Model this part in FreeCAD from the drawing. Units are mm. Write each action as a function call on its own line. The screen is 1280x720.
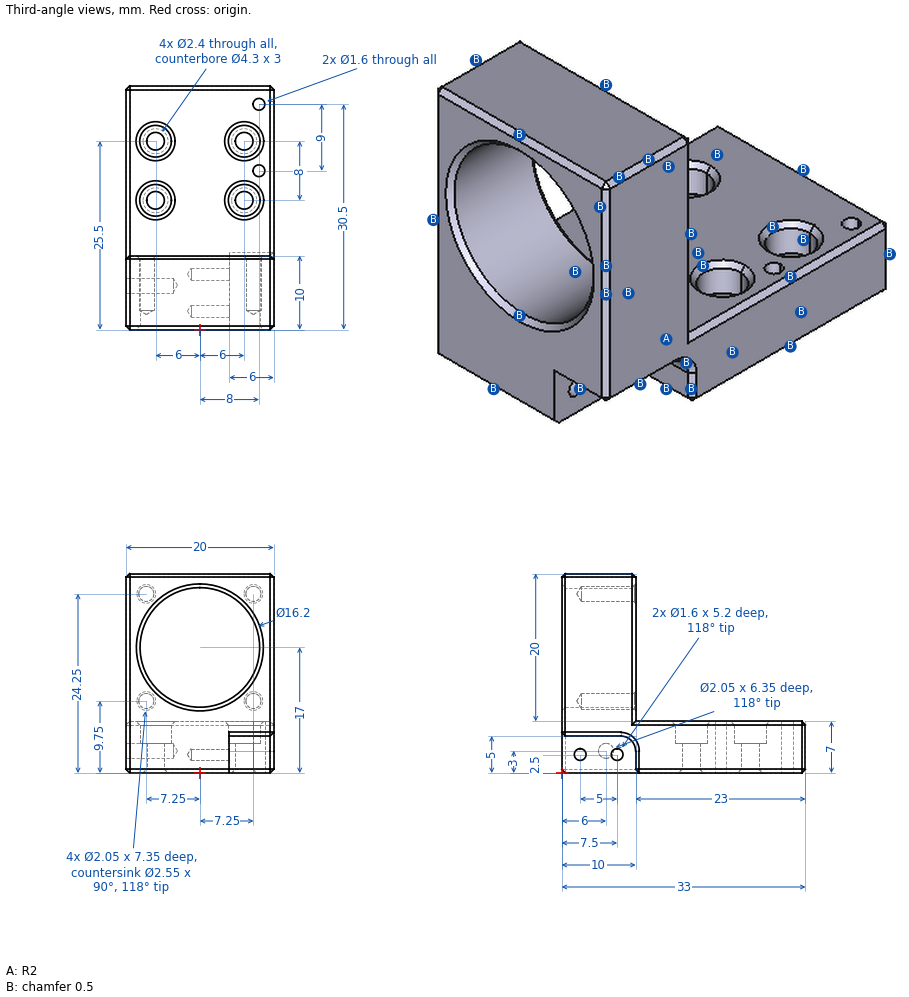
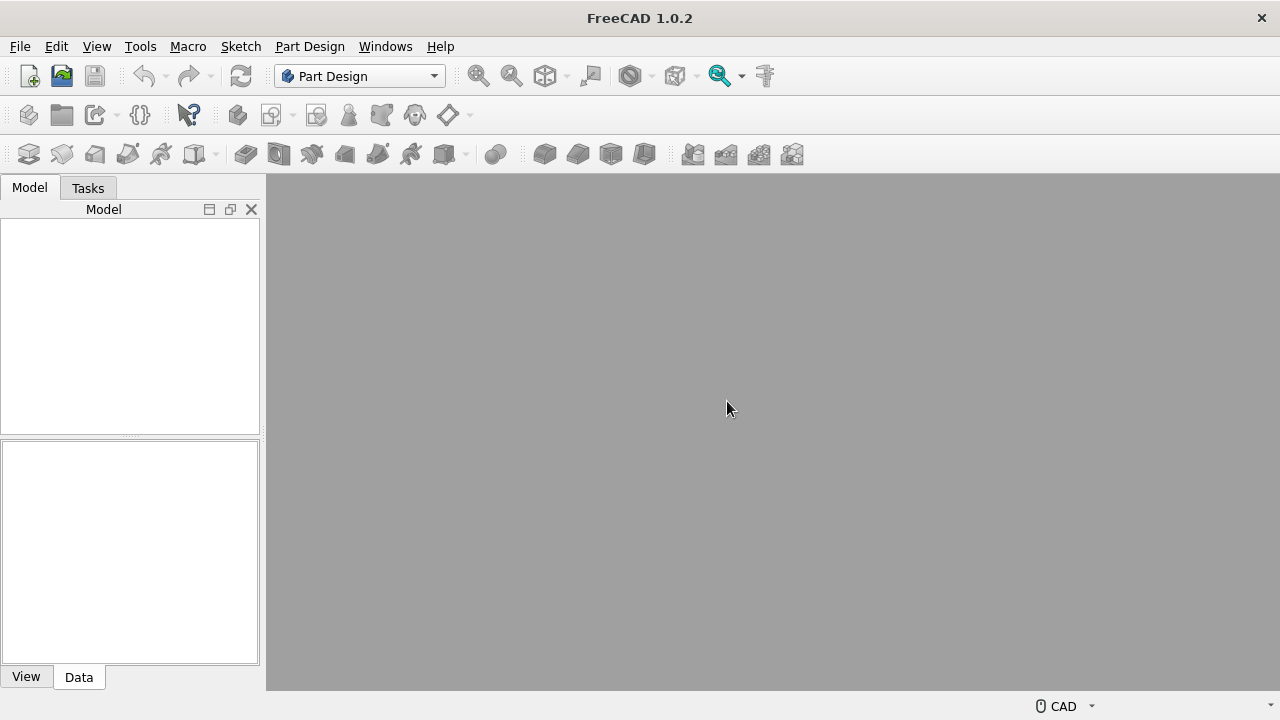
click(29, 76)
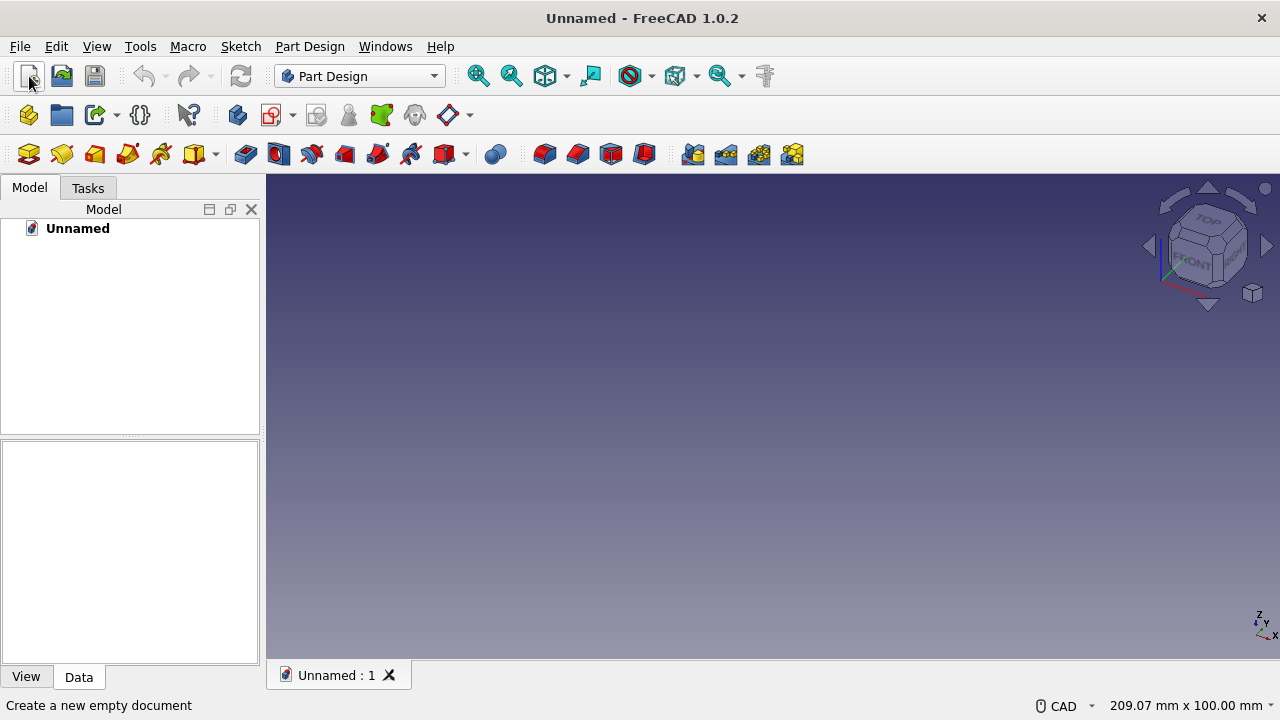
click(270, 116)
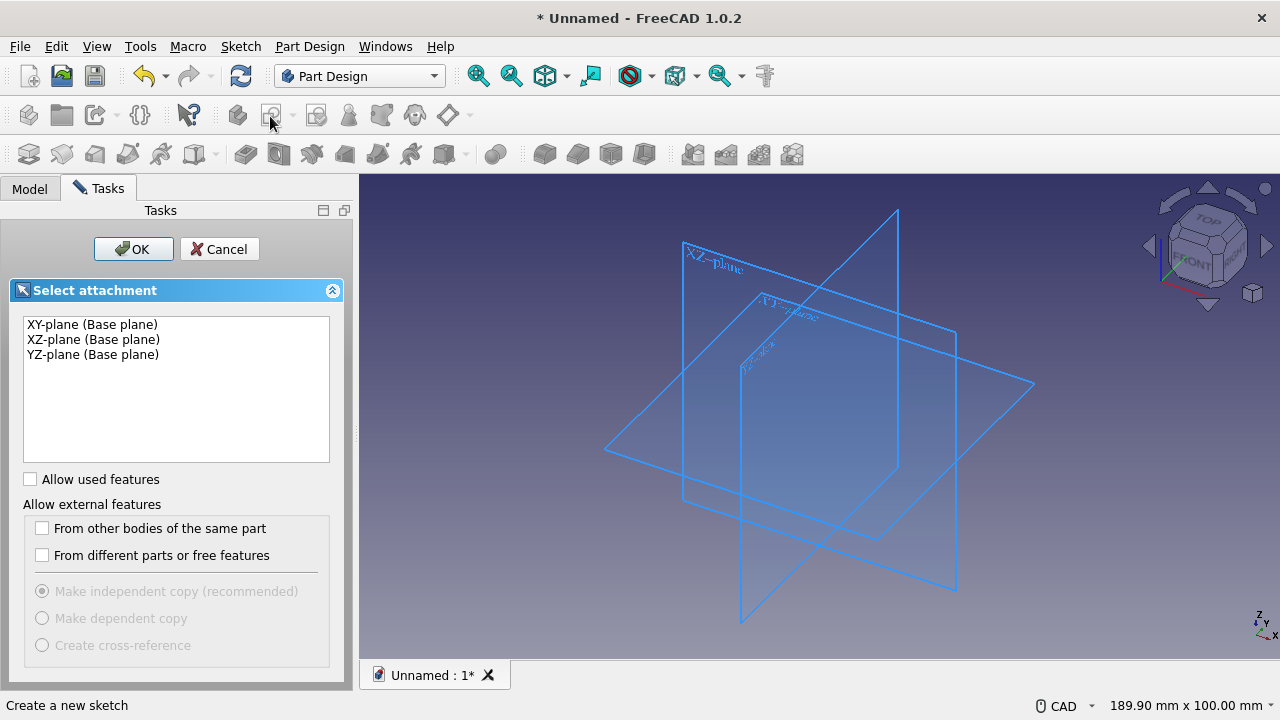
click(84, 354)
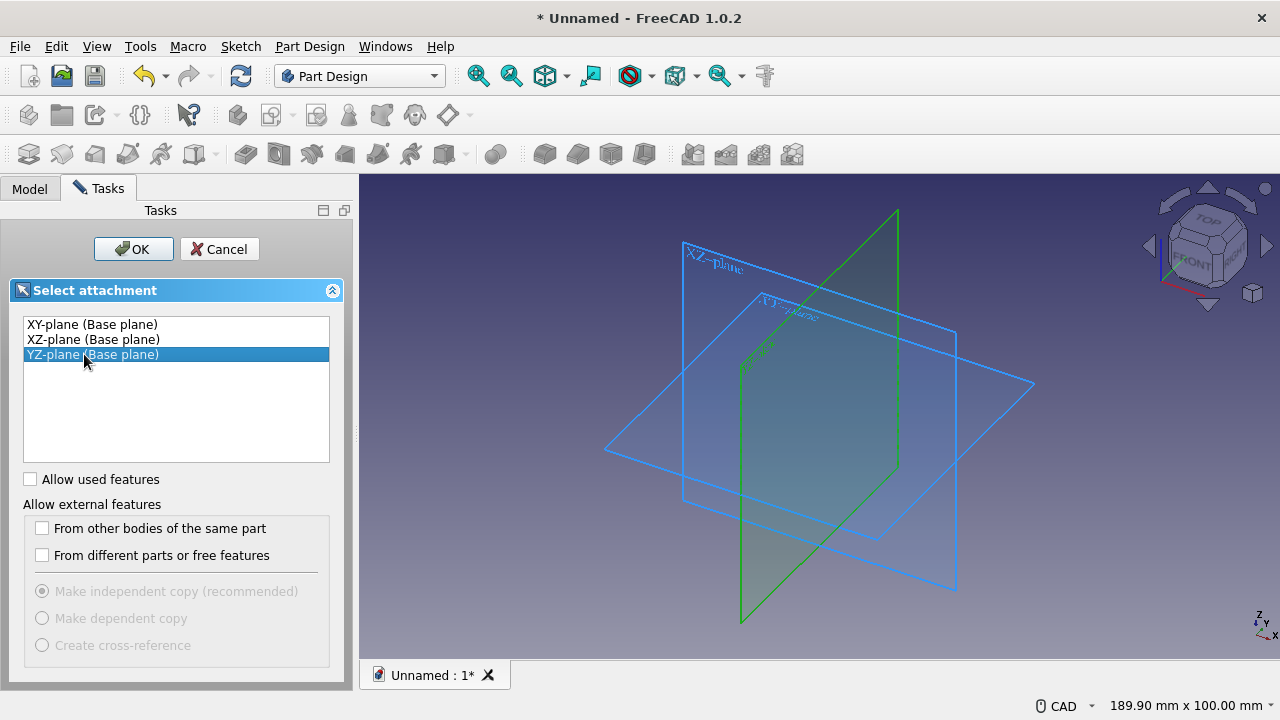
click(134, 249)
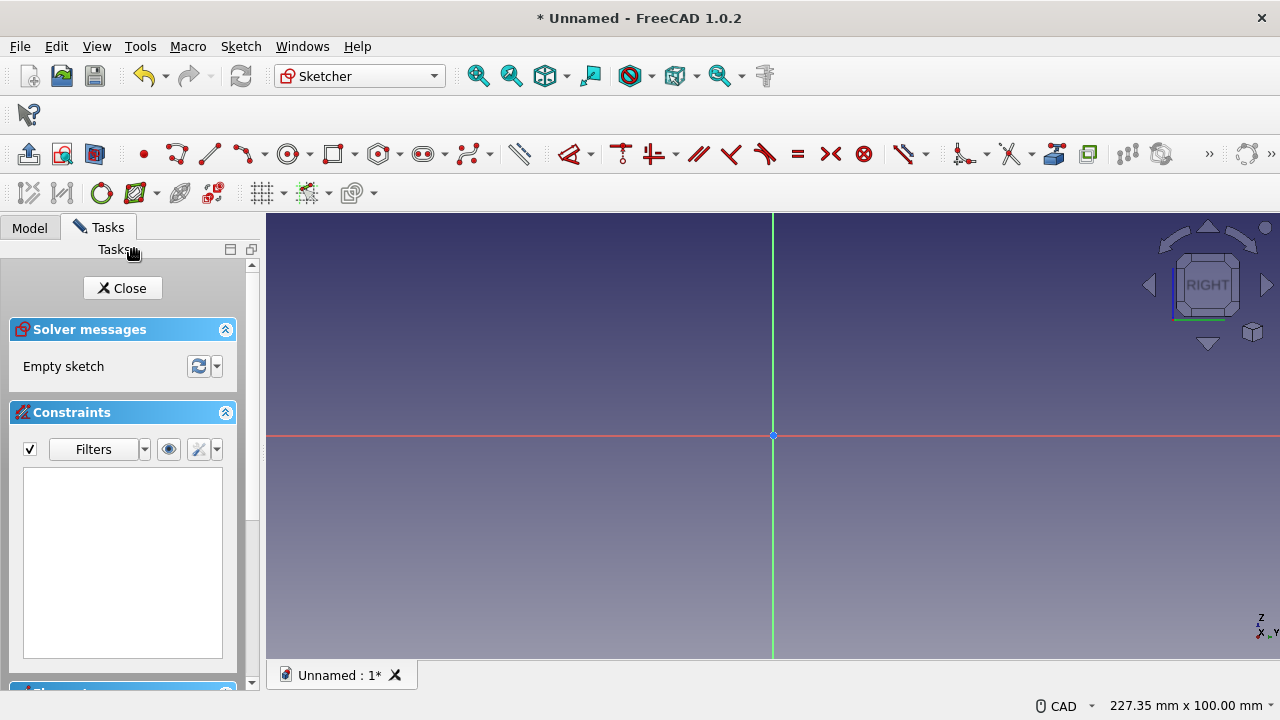
scroll(963, 327, up, 4)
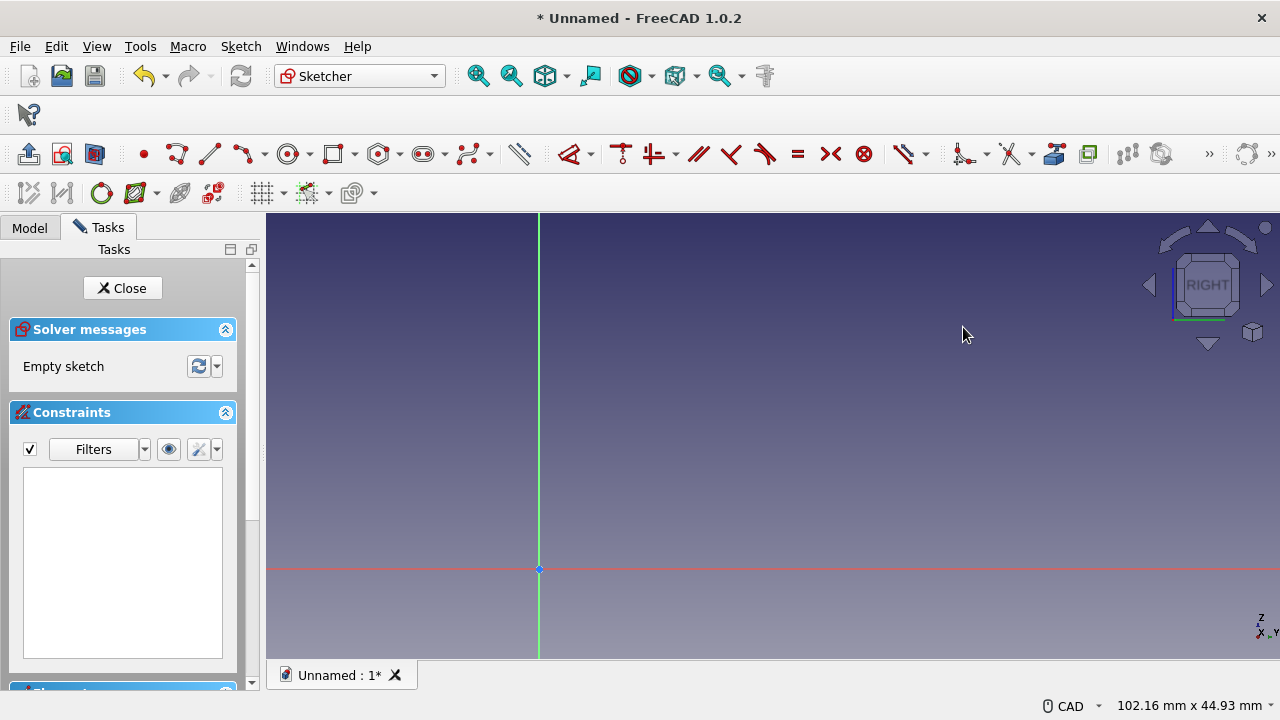
click(177, 154)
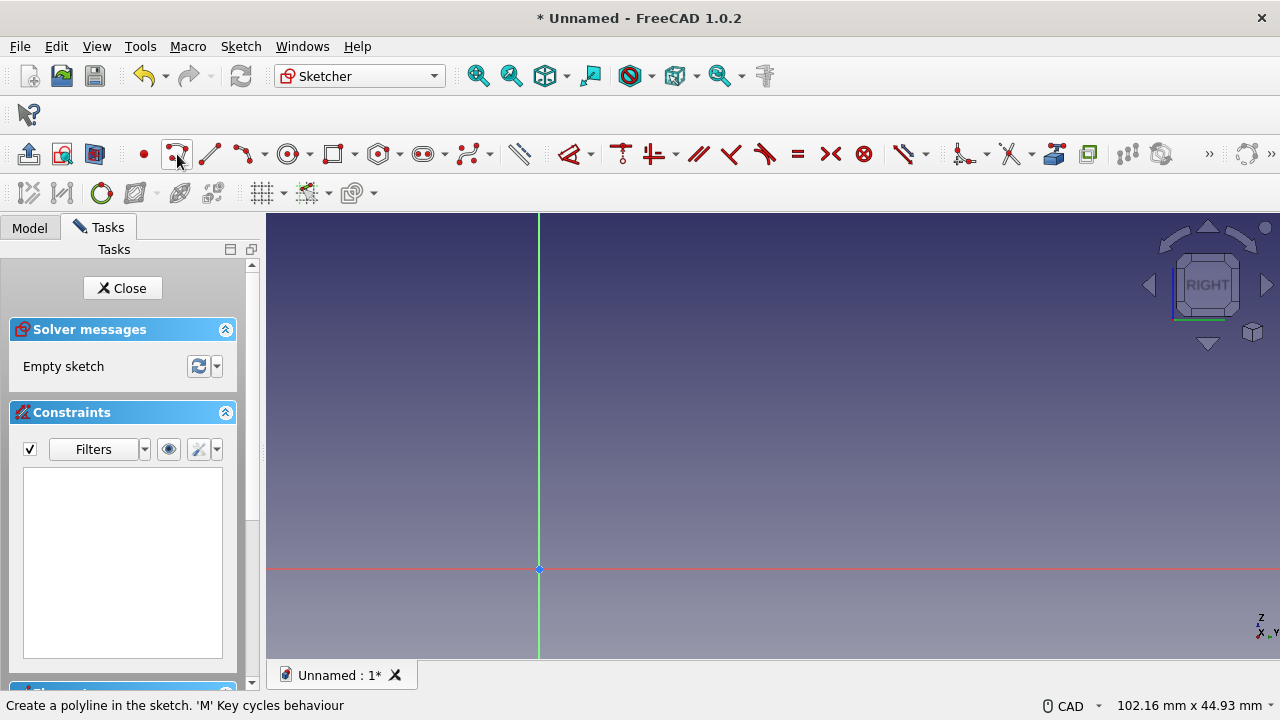
click(539, 569)
click(867, 560)
click(867, 500)
click(639, 500)
click(639, 301)
click(548, 301)
click(539, 569)
key(Escape)
key(Escape)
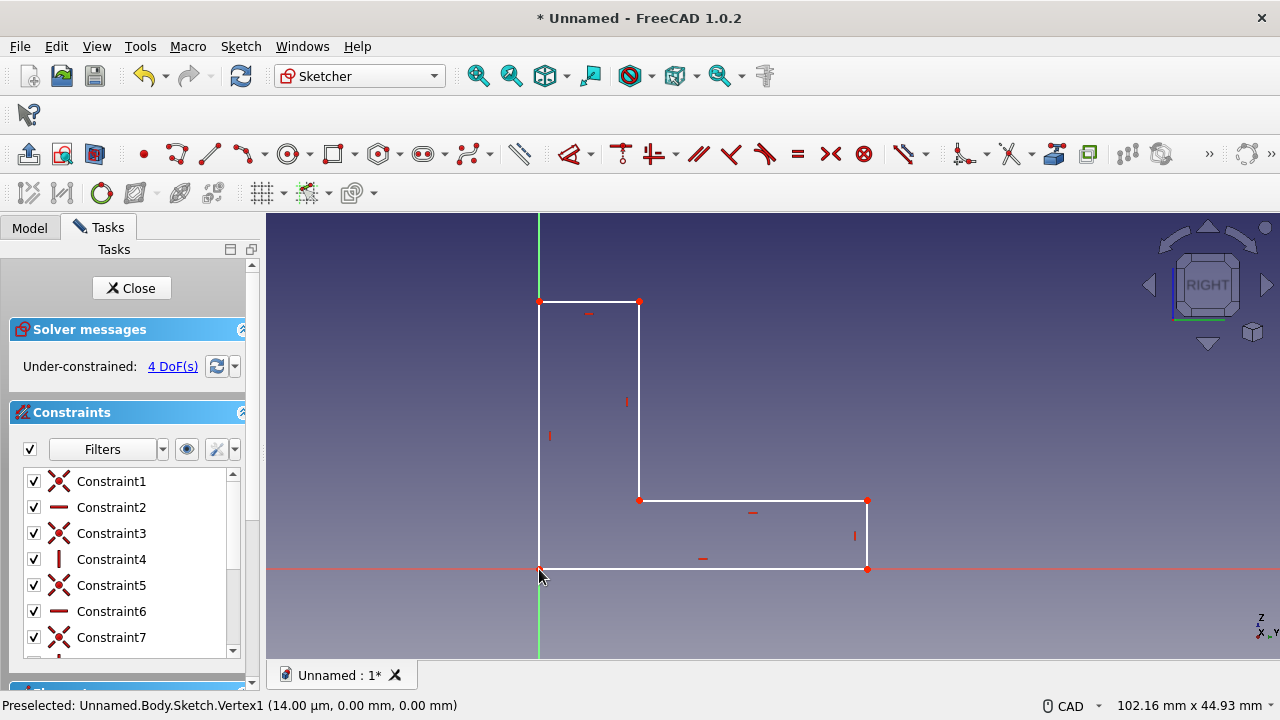
key(d)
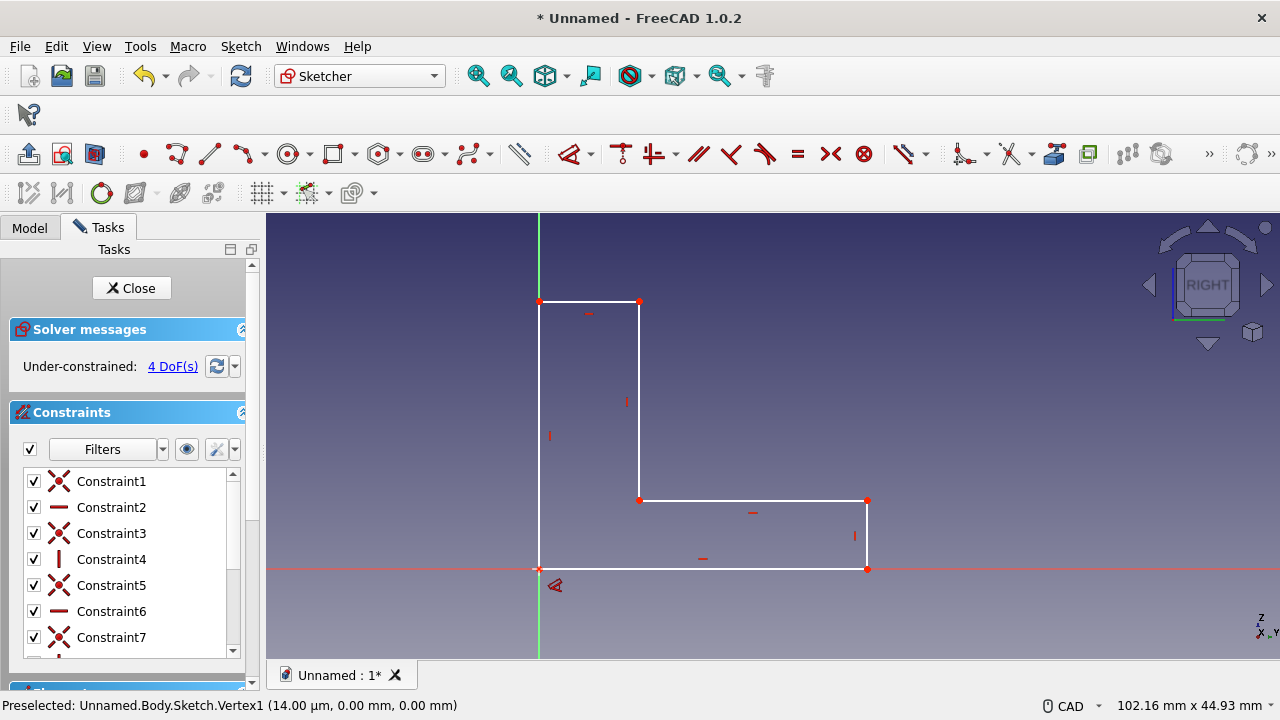
click(867, 549)
click(901, 535)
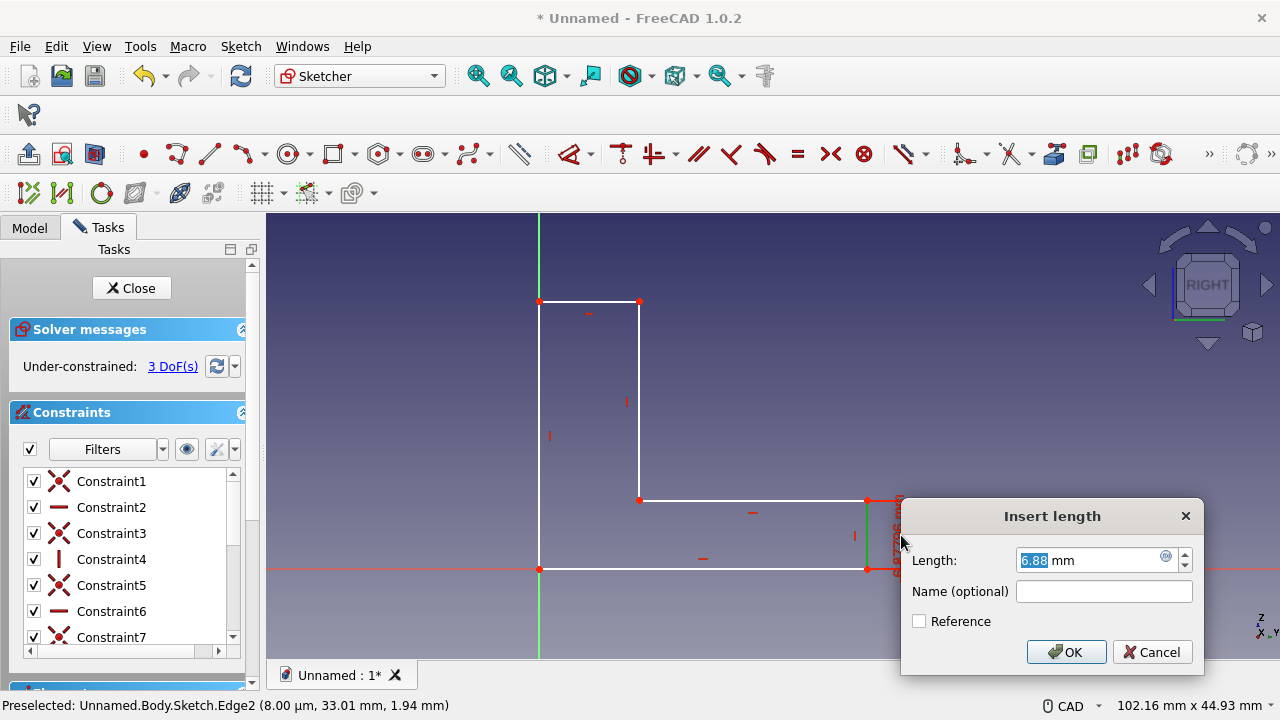
text(7)
key(Return)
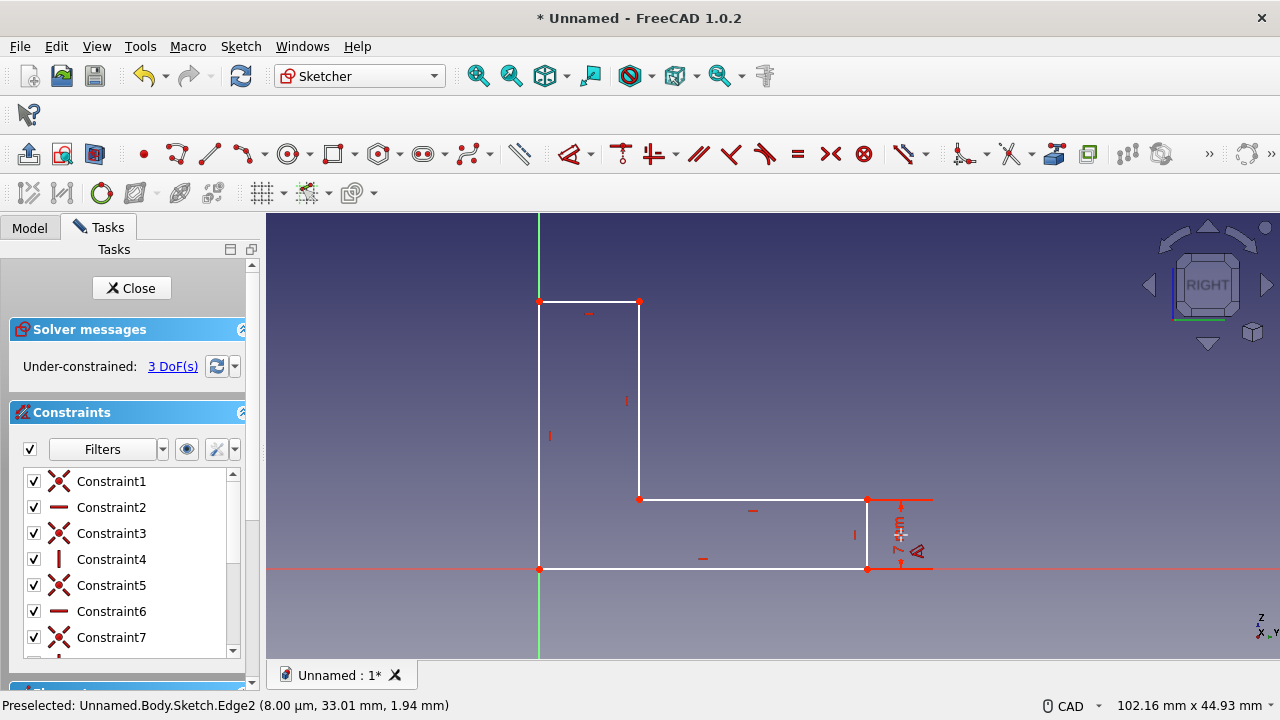
click(638, 569)
click(703, 603)